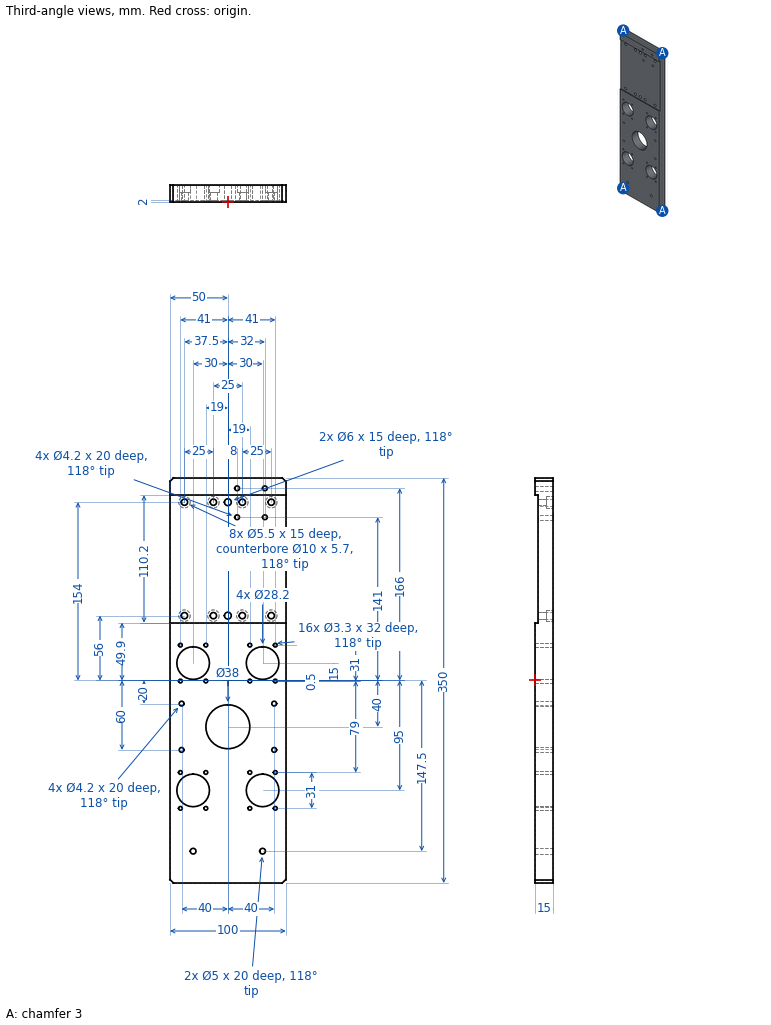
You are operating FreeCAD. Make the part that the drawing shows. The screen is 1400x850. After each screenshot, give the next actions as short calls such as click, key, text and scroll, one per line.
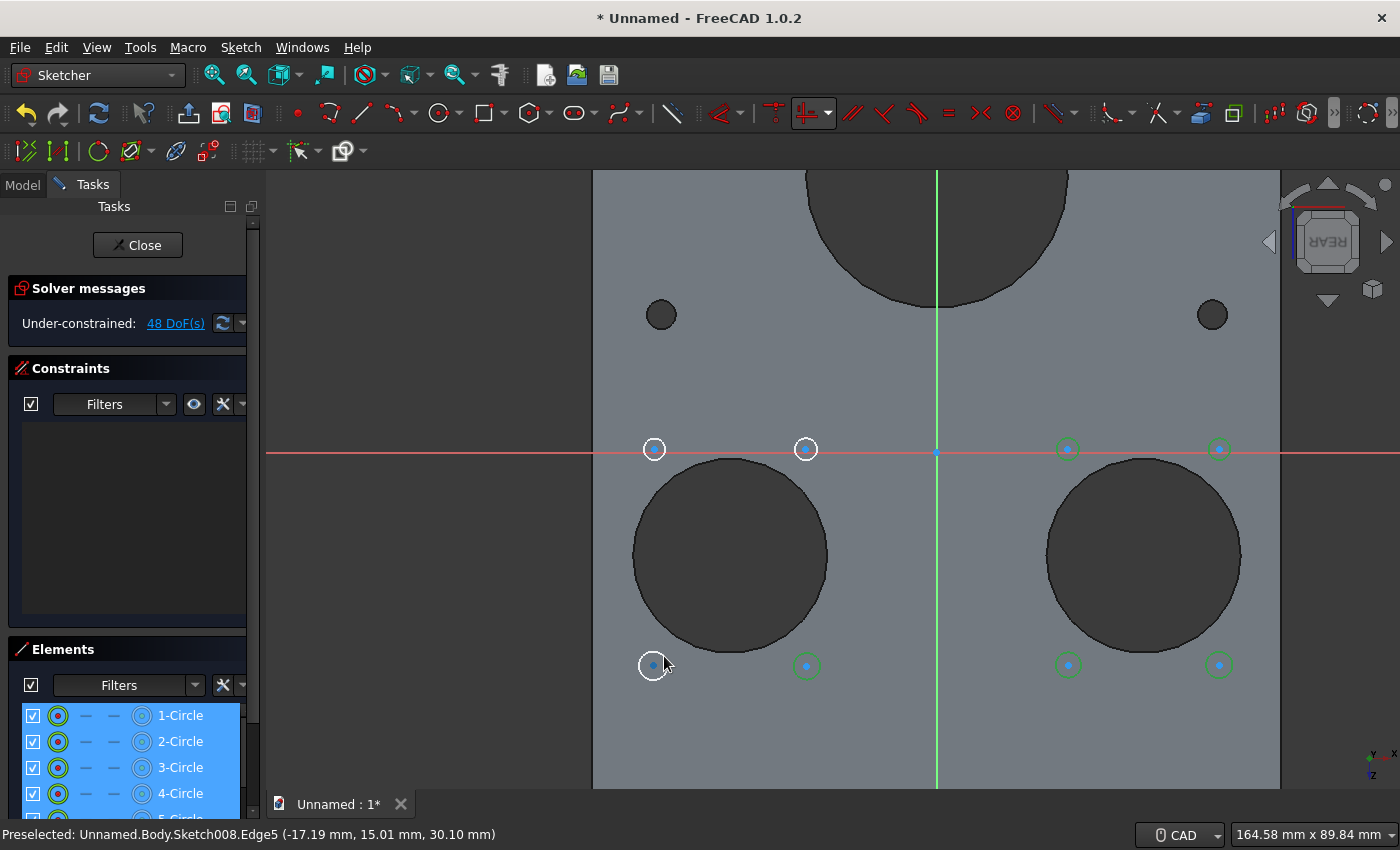
click(663, 656)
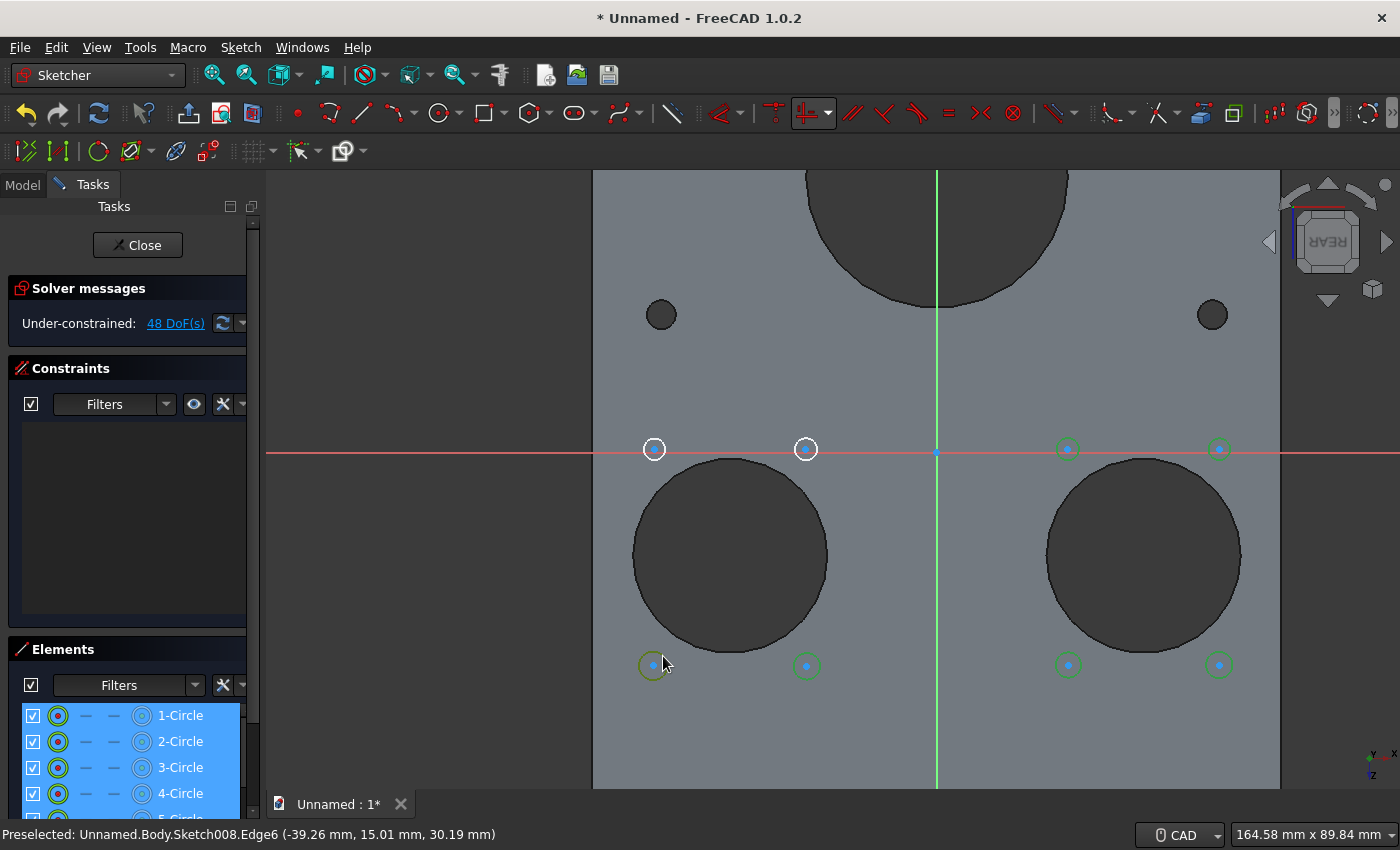
scroll(814, 441, up, 2)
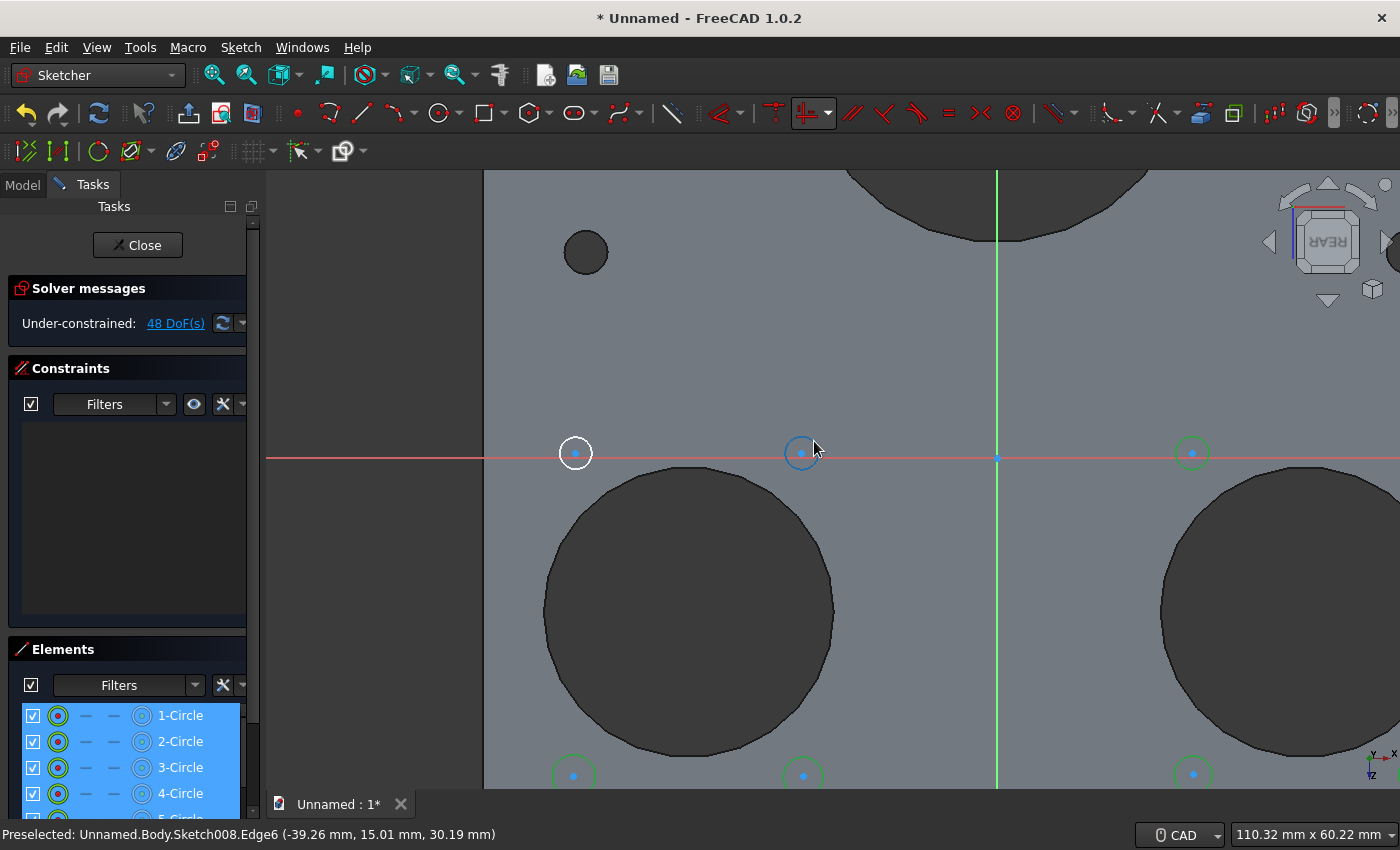
click(813, 442)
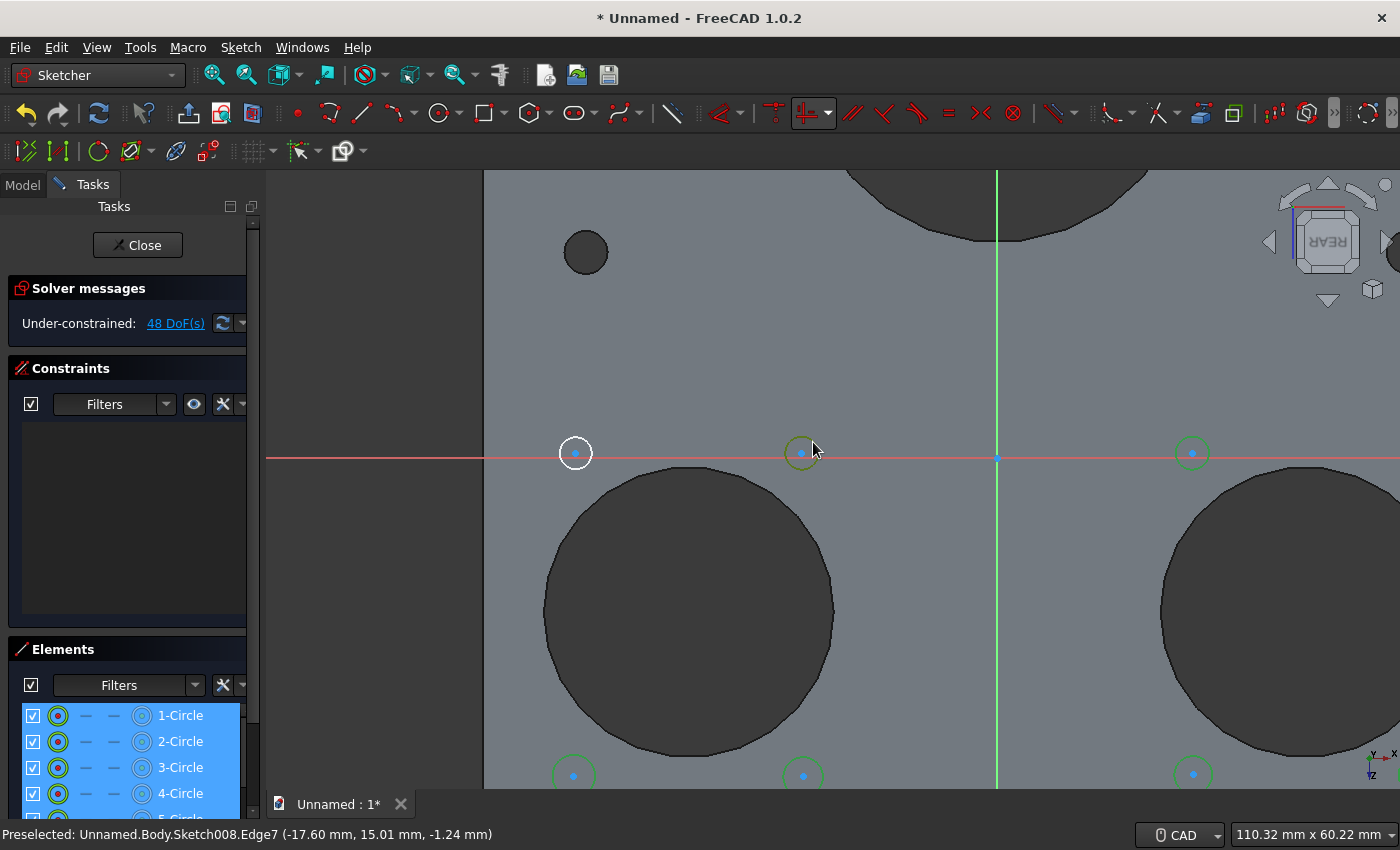
click(587, 442)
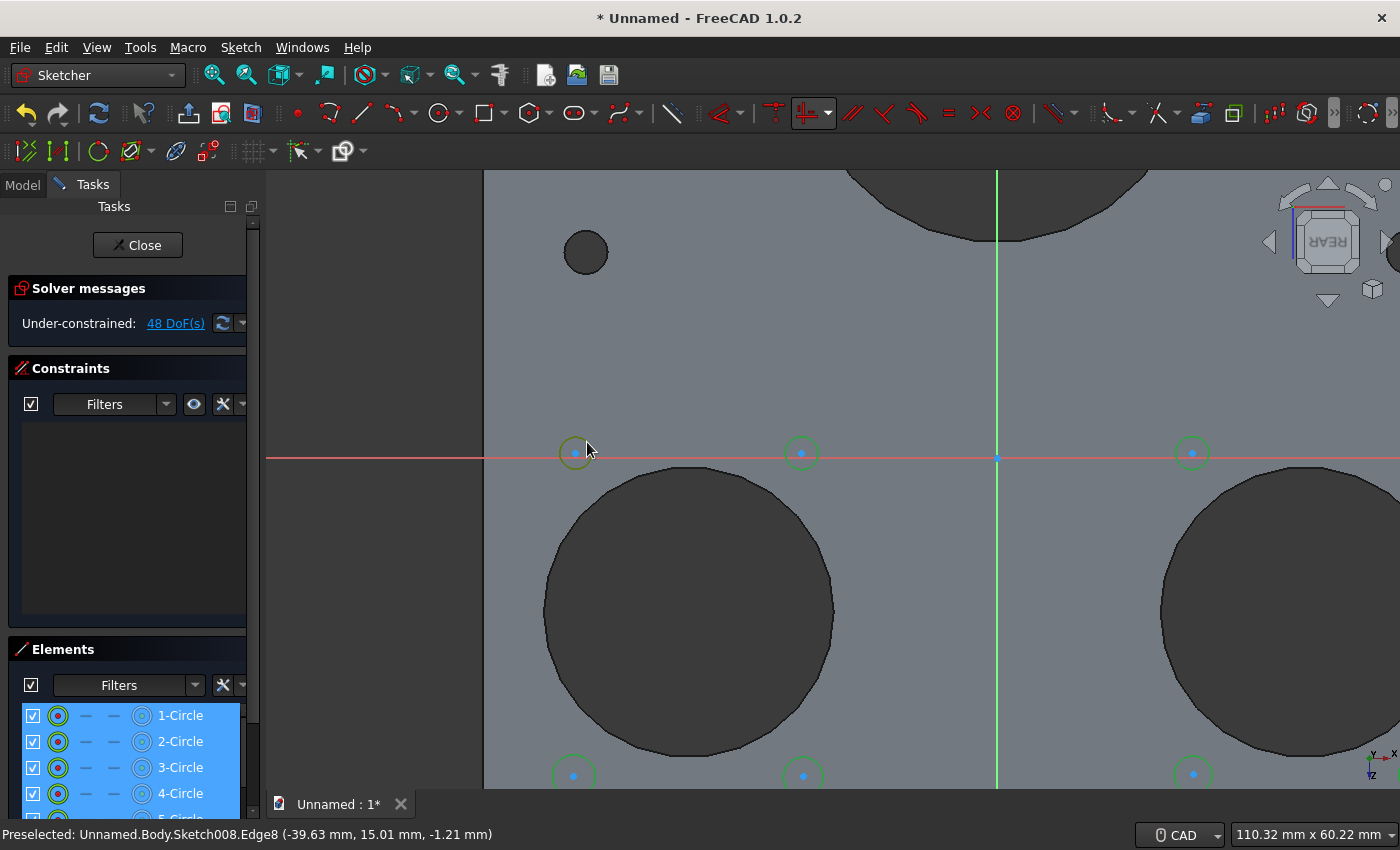
scroll(688, 621, down, 7)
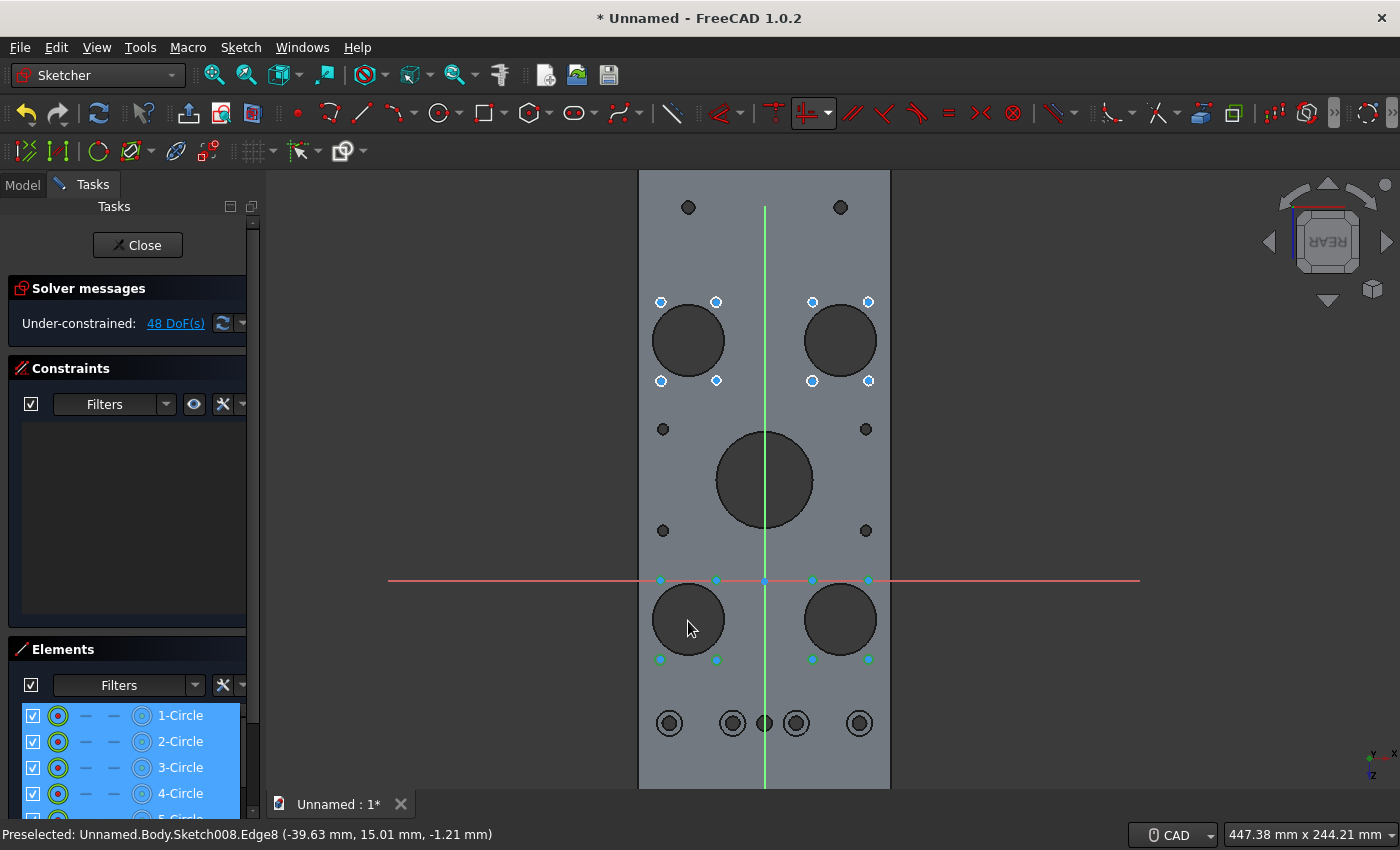
scroll(872, 378, up, 6)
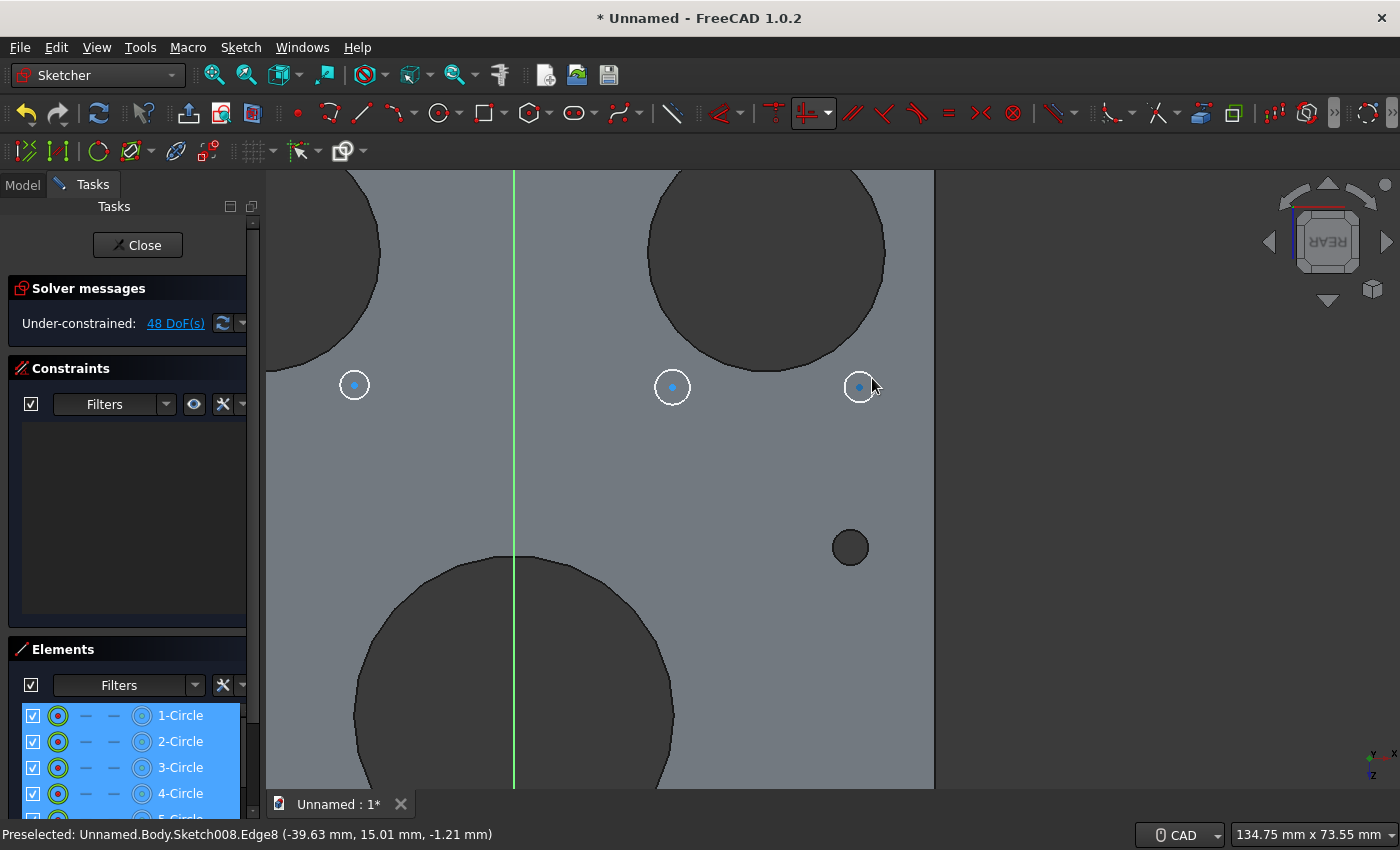
click(871, 376)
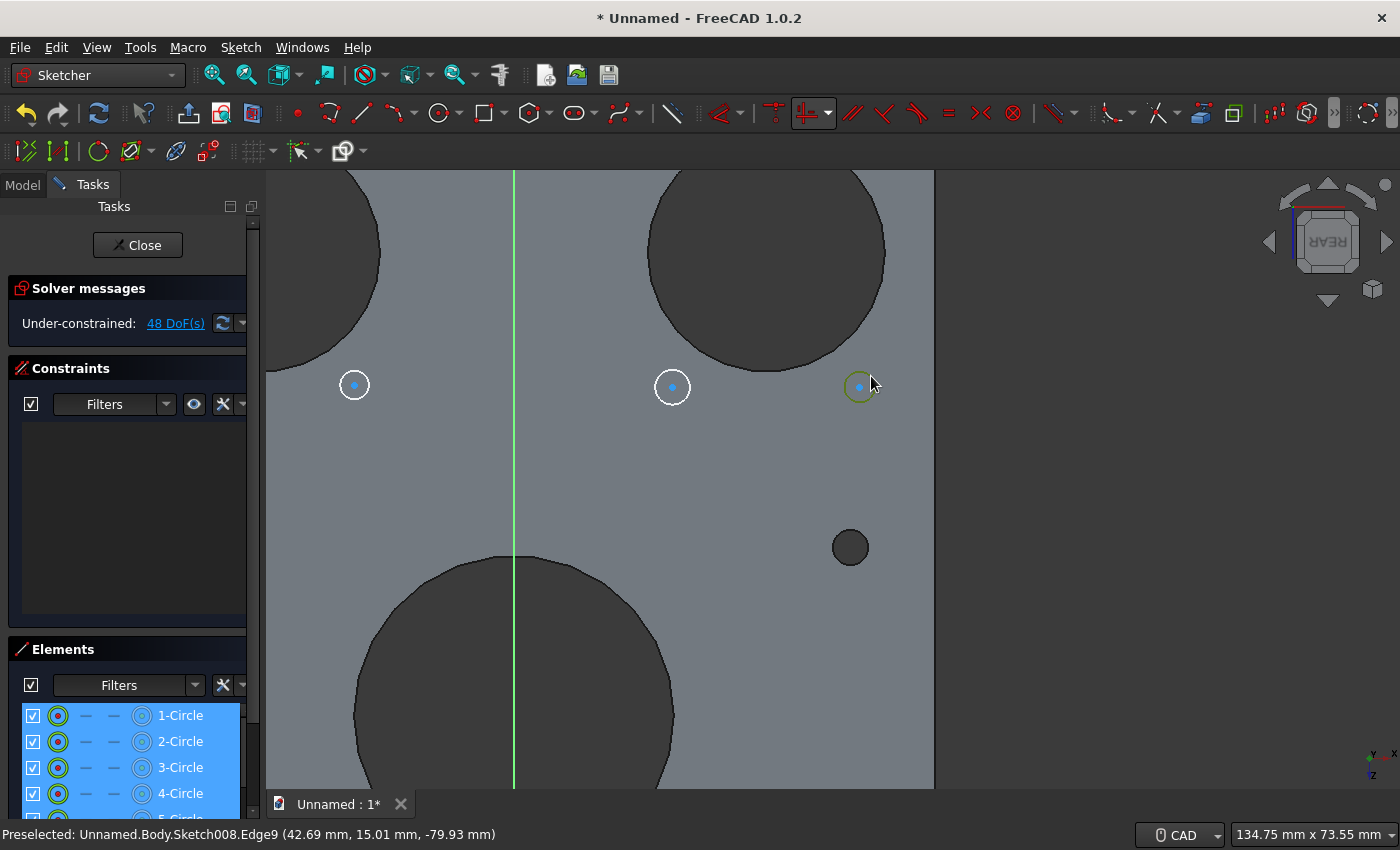
click(685, 375)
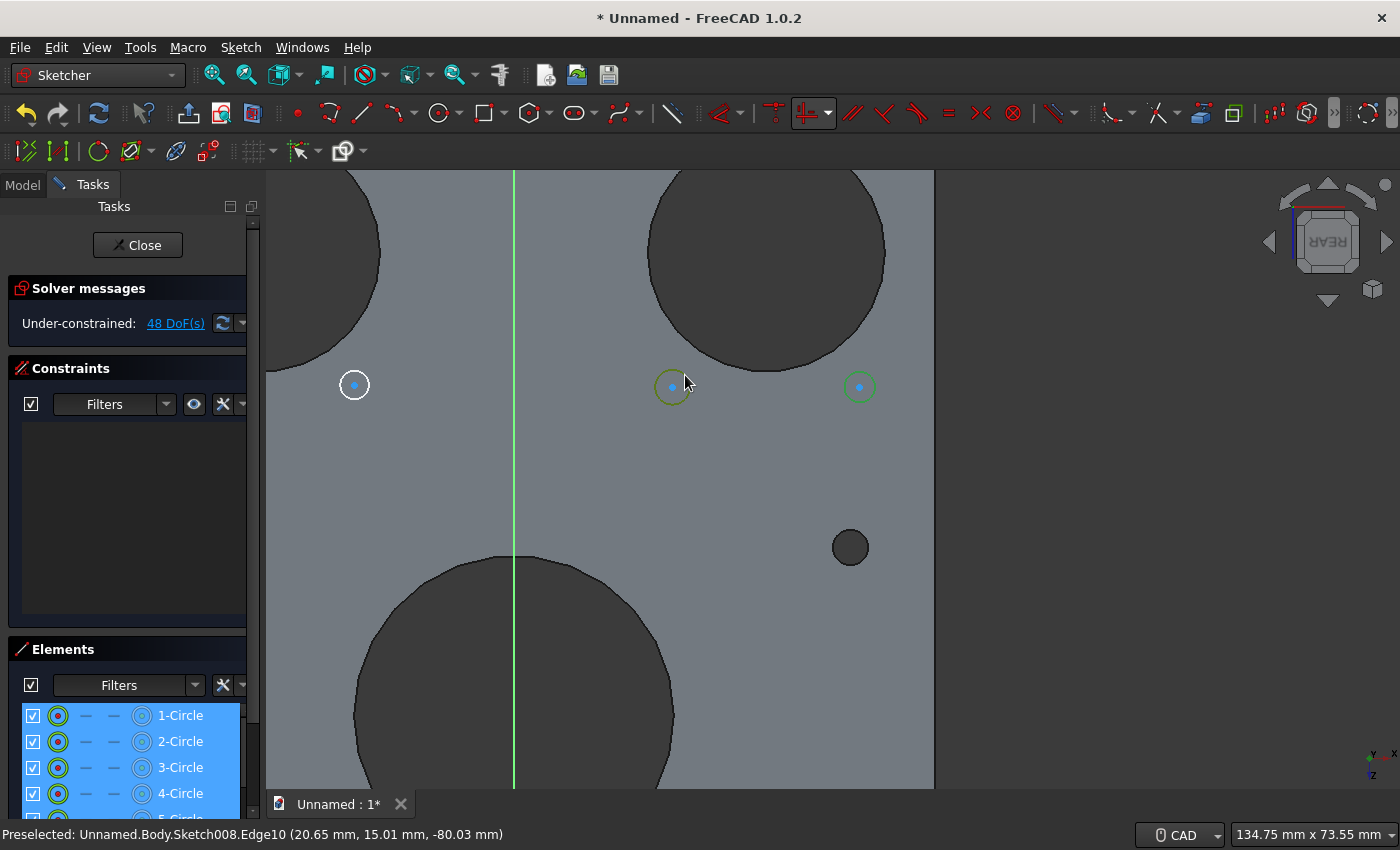
scroll(873, 378, down, 6)